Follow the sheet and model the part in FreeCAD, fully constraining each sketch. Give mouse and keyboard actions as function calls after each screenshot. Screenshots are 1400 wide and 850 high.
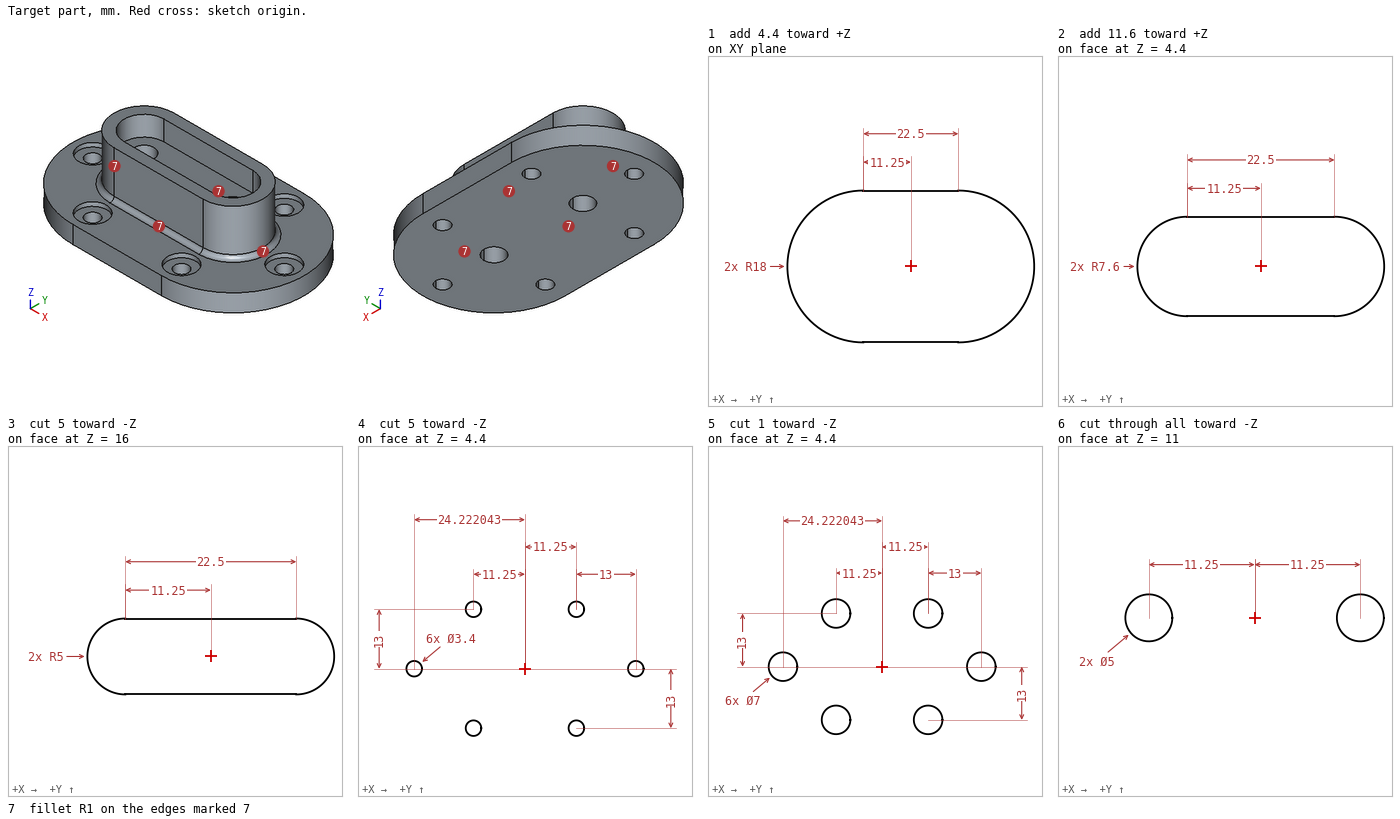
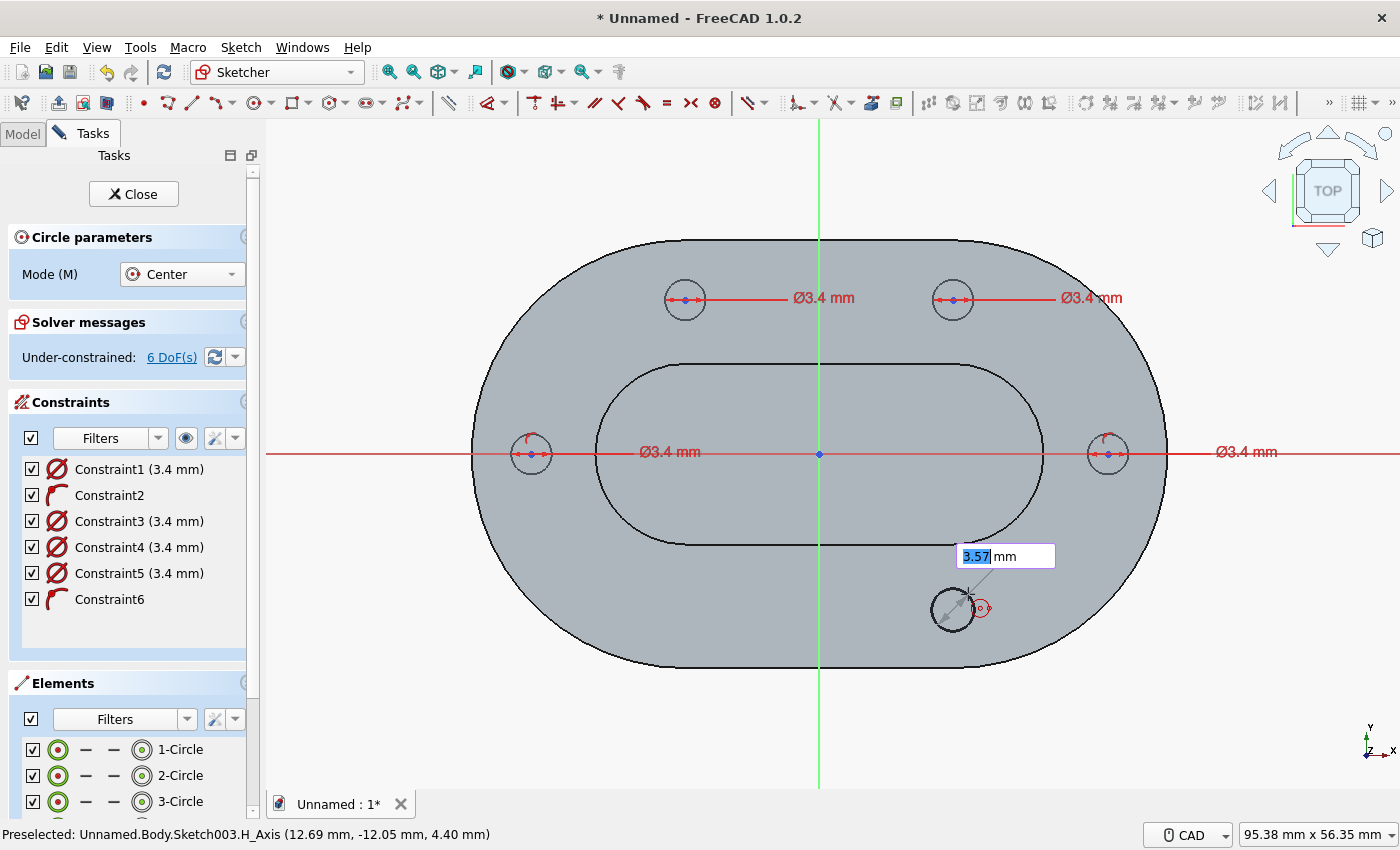
text(3.4)
key(Return)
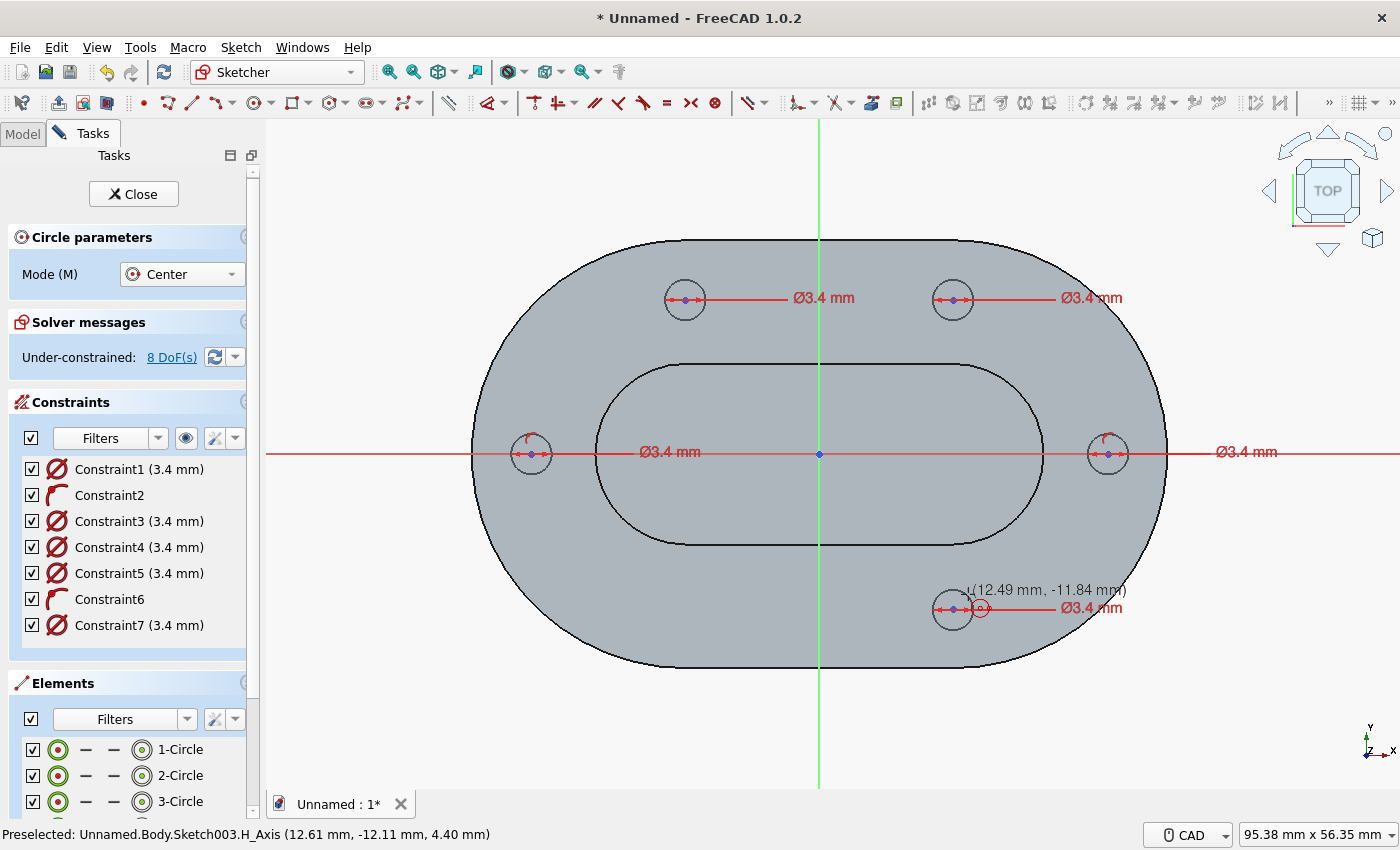
click(686, 609)
move(700, 594)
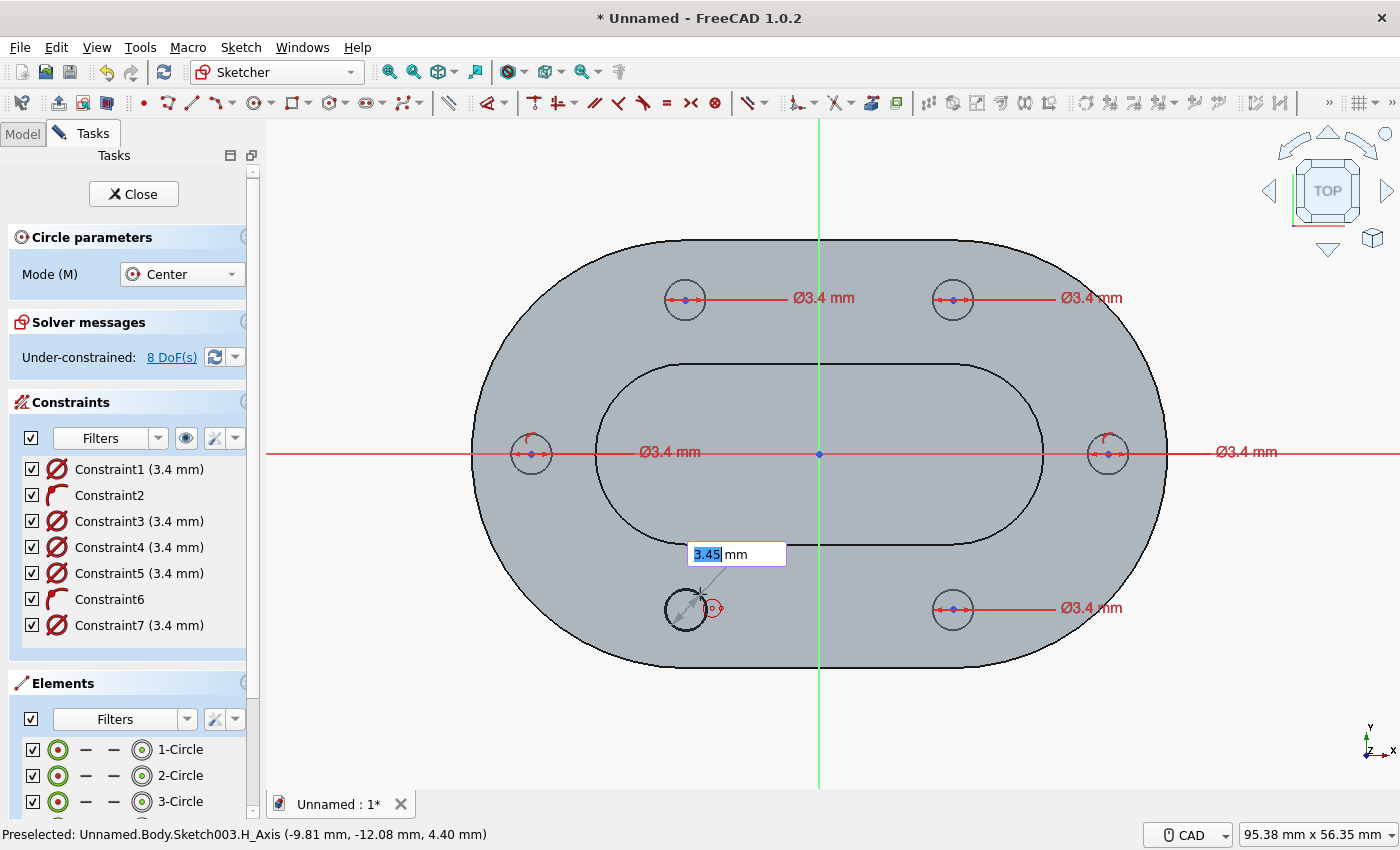
text(3.4)
key(Return)
key(Escape)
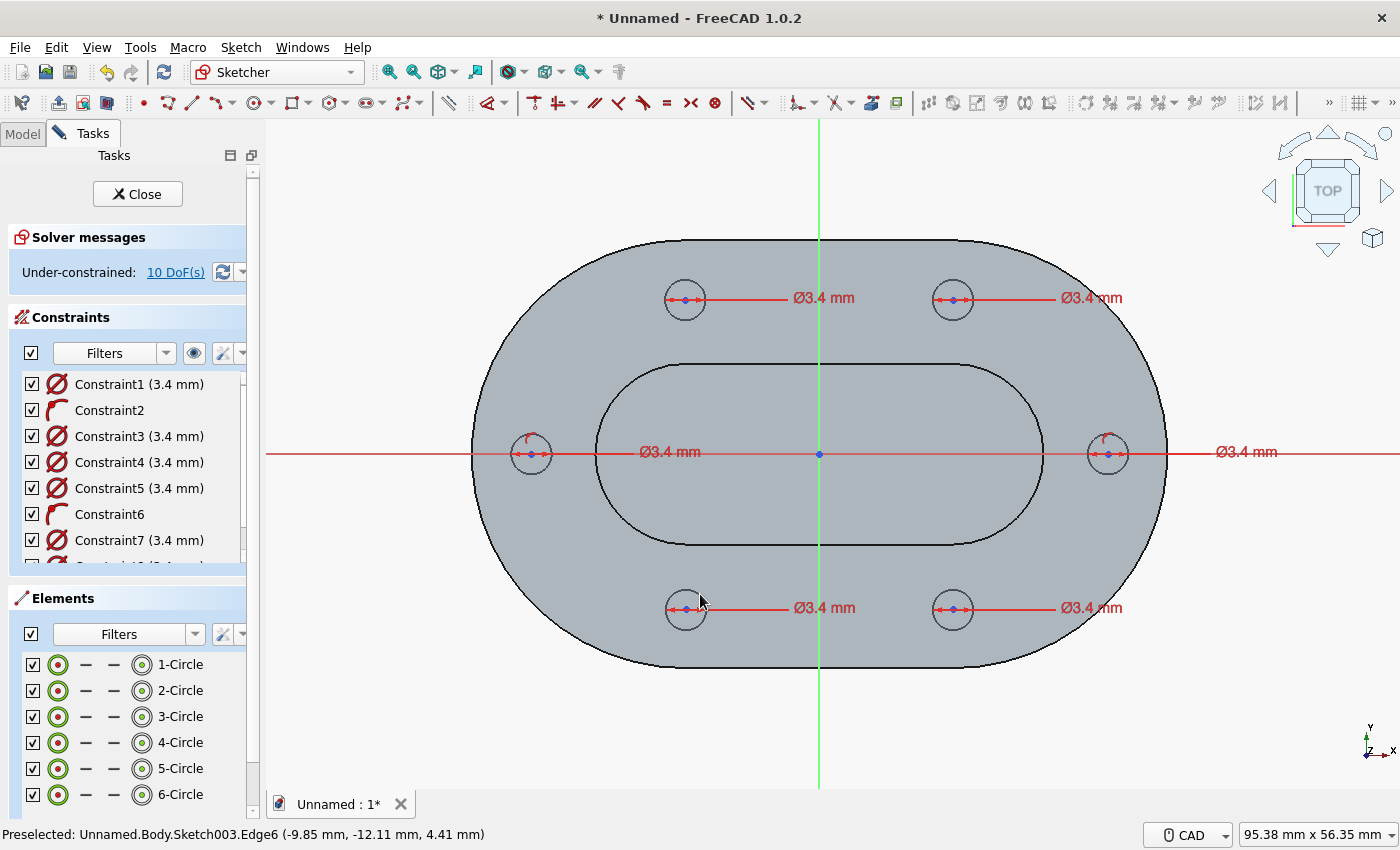
click(685, 300)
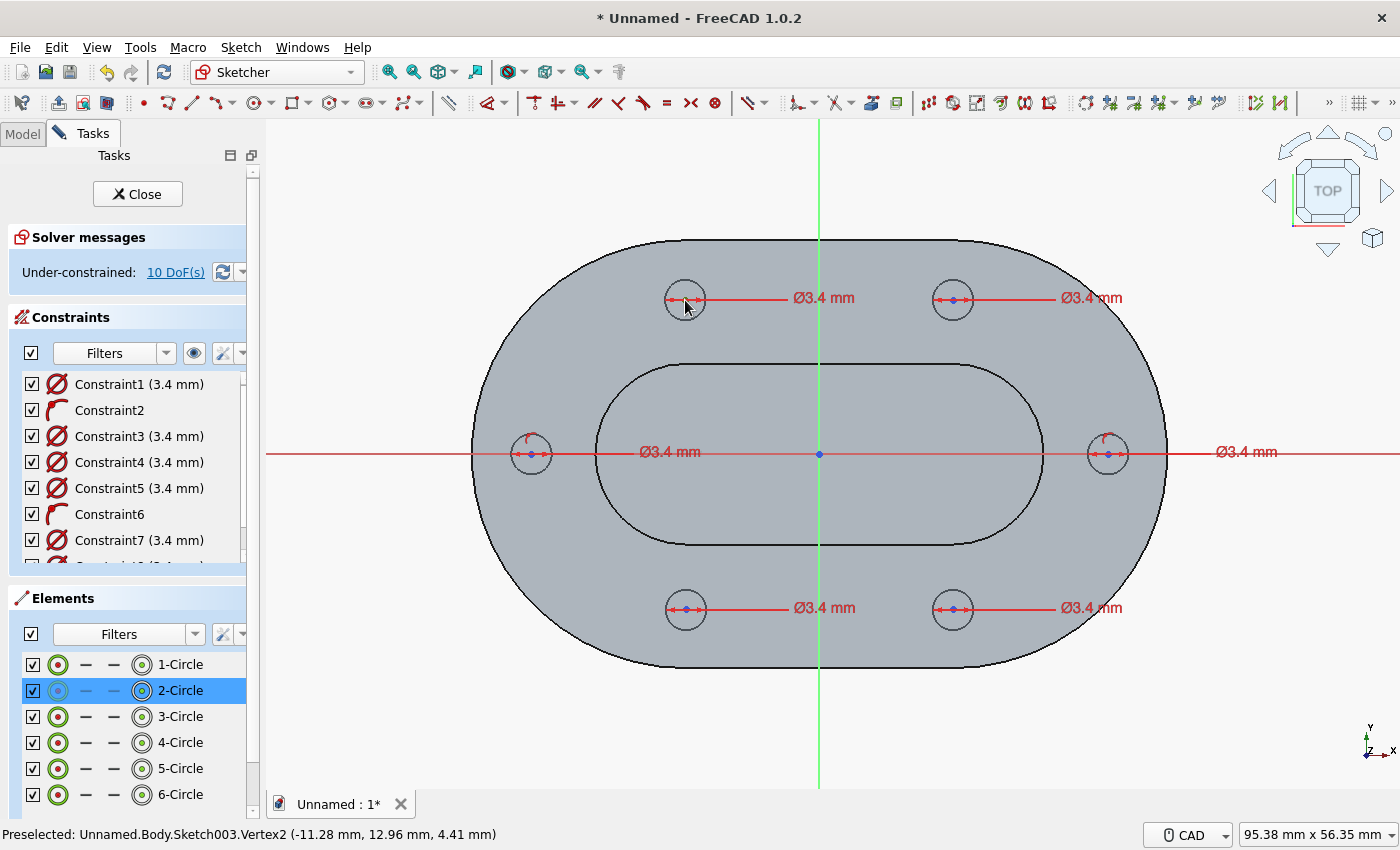
click(953, 300)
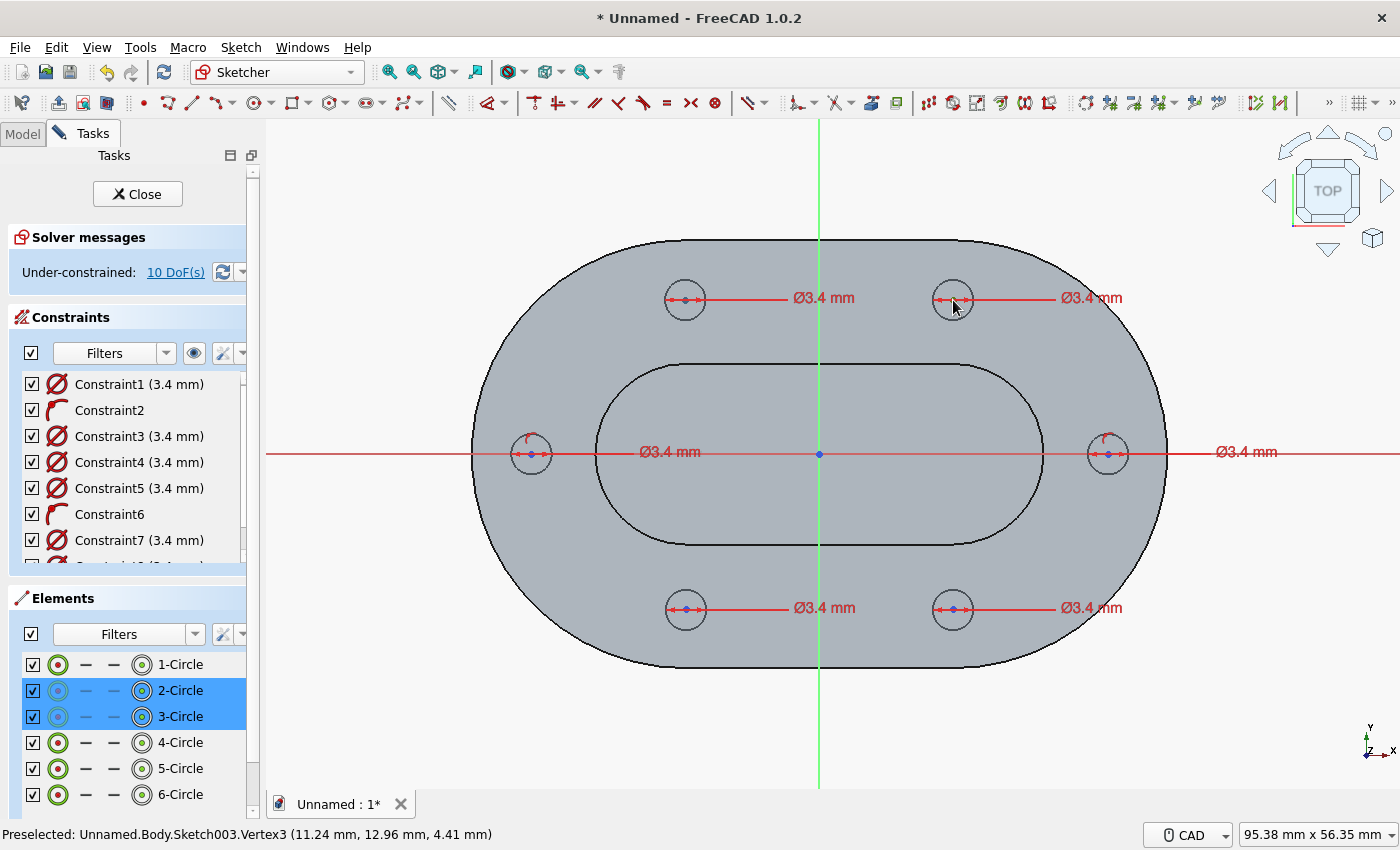
click(576, 104)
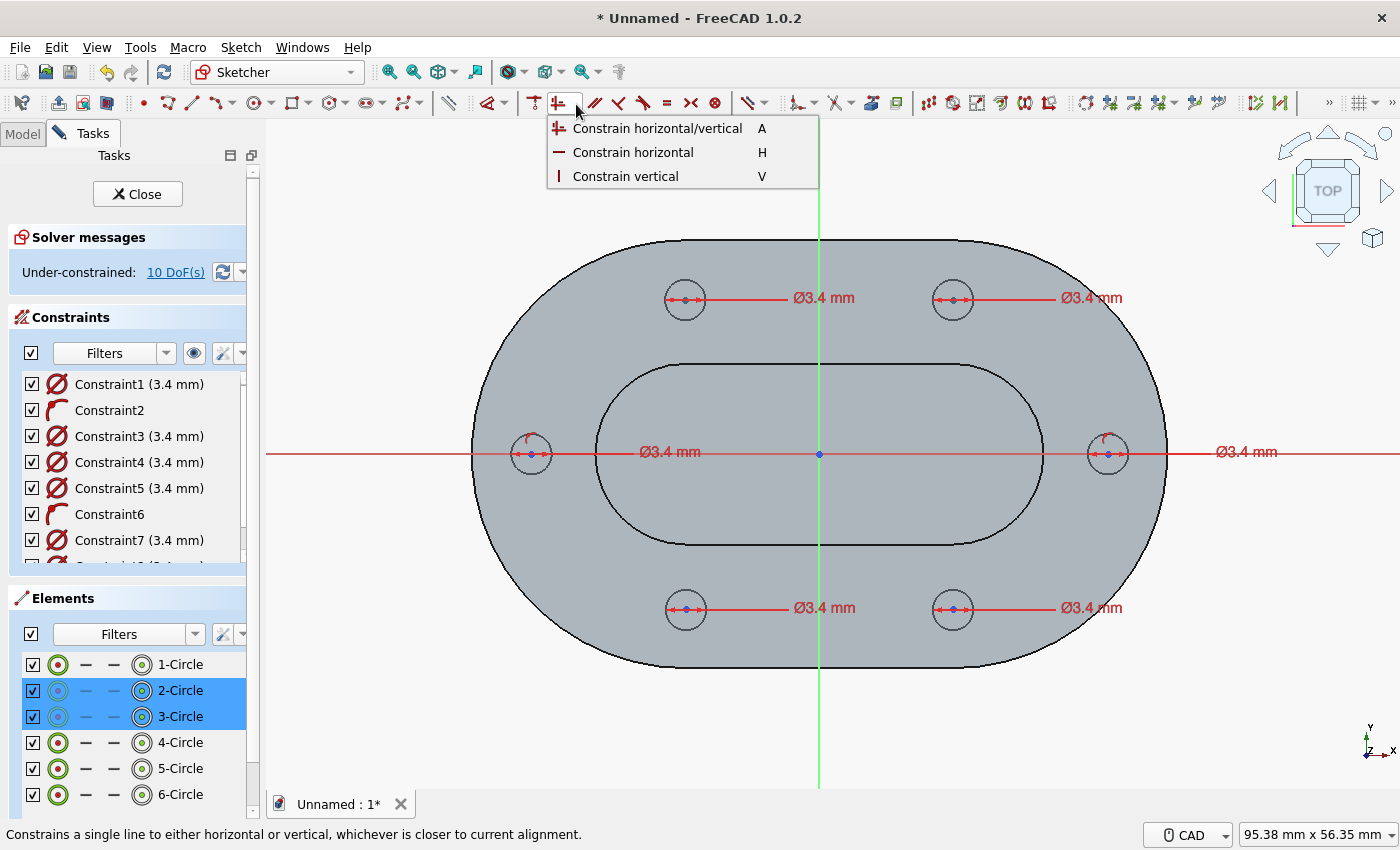
click(683, 152)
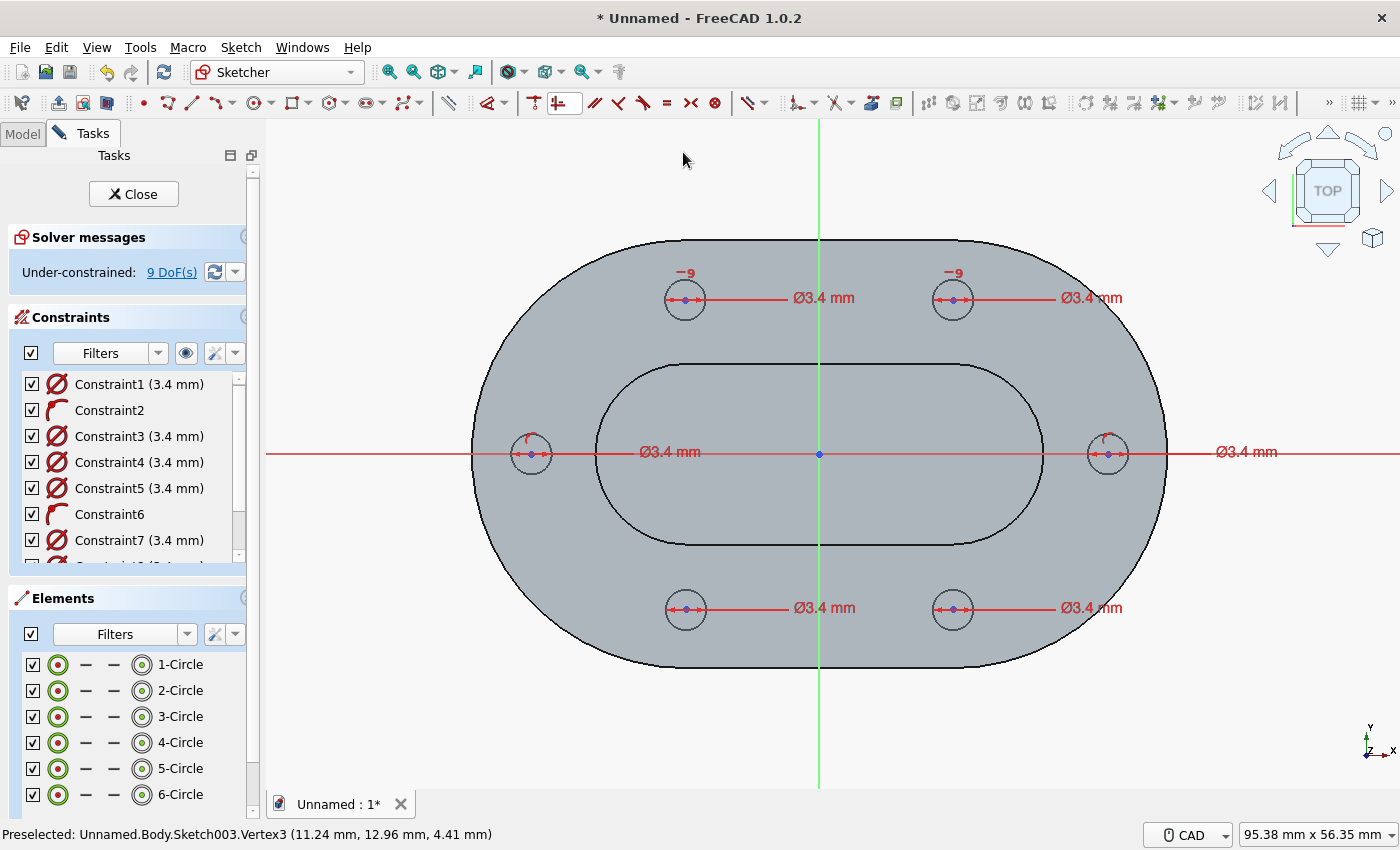
click(953, 300)